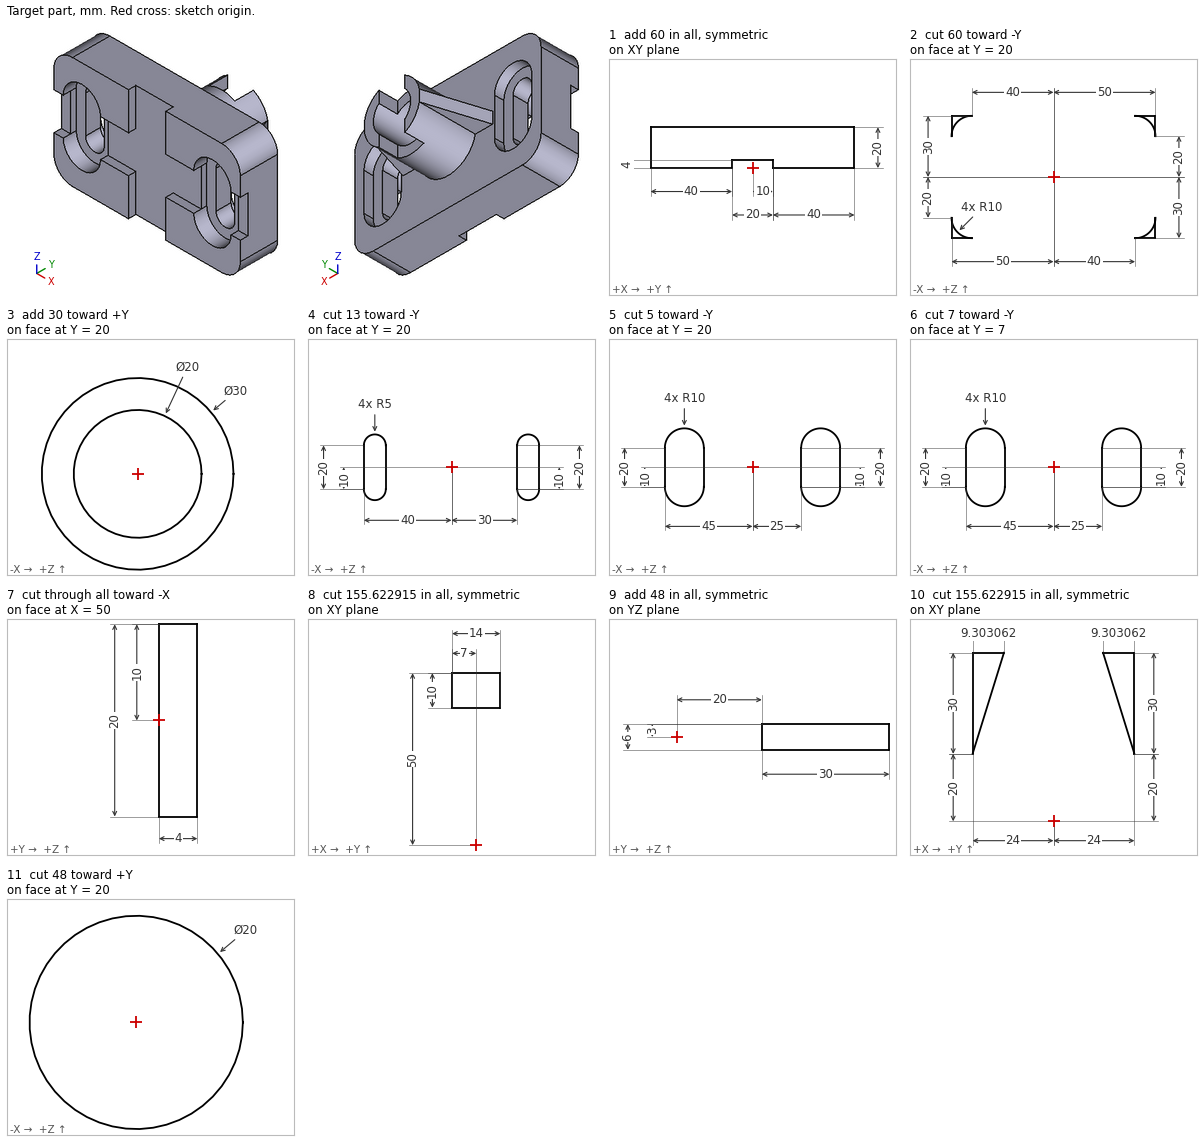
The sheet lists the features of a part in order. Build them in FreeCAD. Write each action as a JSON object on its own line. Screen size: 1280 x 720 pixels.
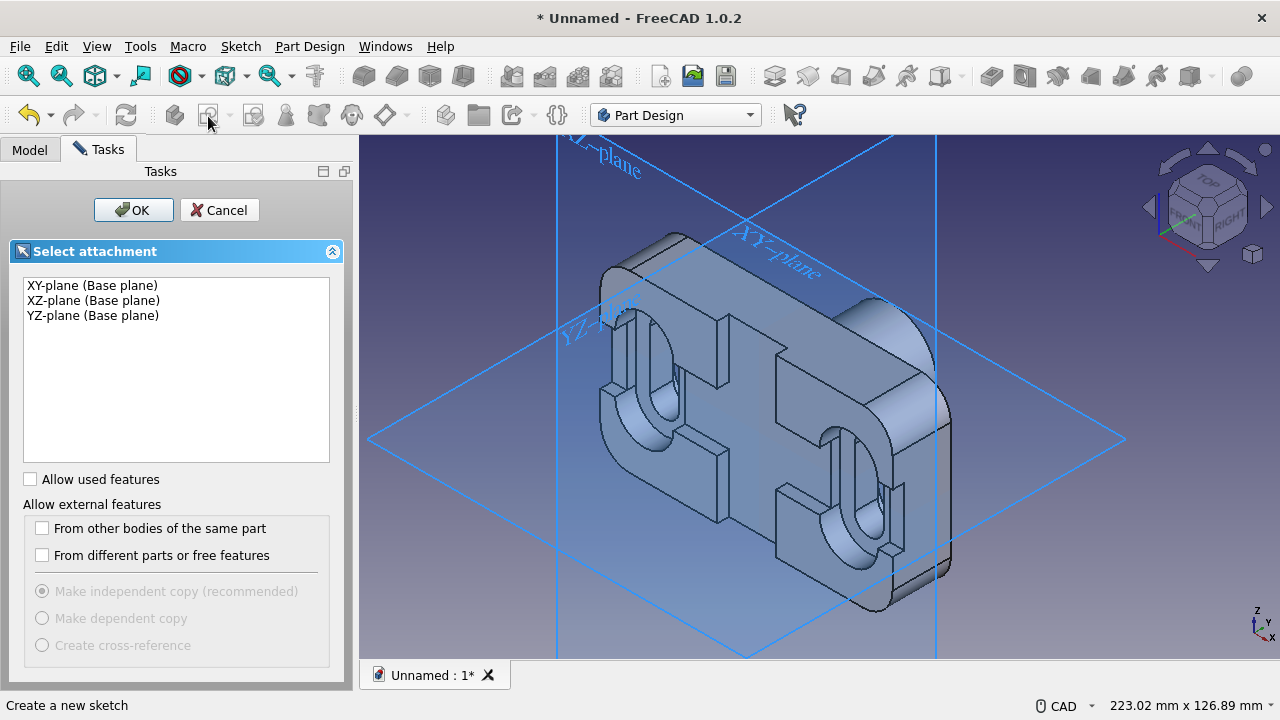
{"action": "left_click", "coordinate": [84, 286]}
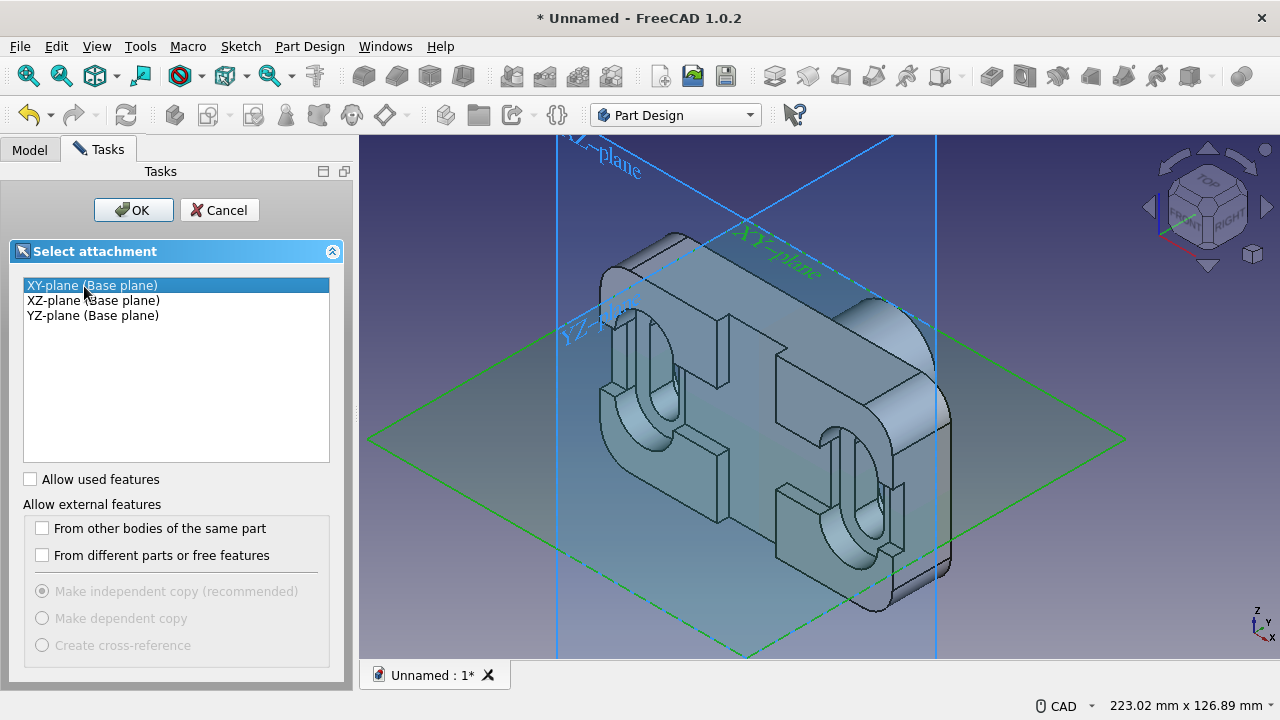
{"action": "left_click", "coordinate": [134, 210]}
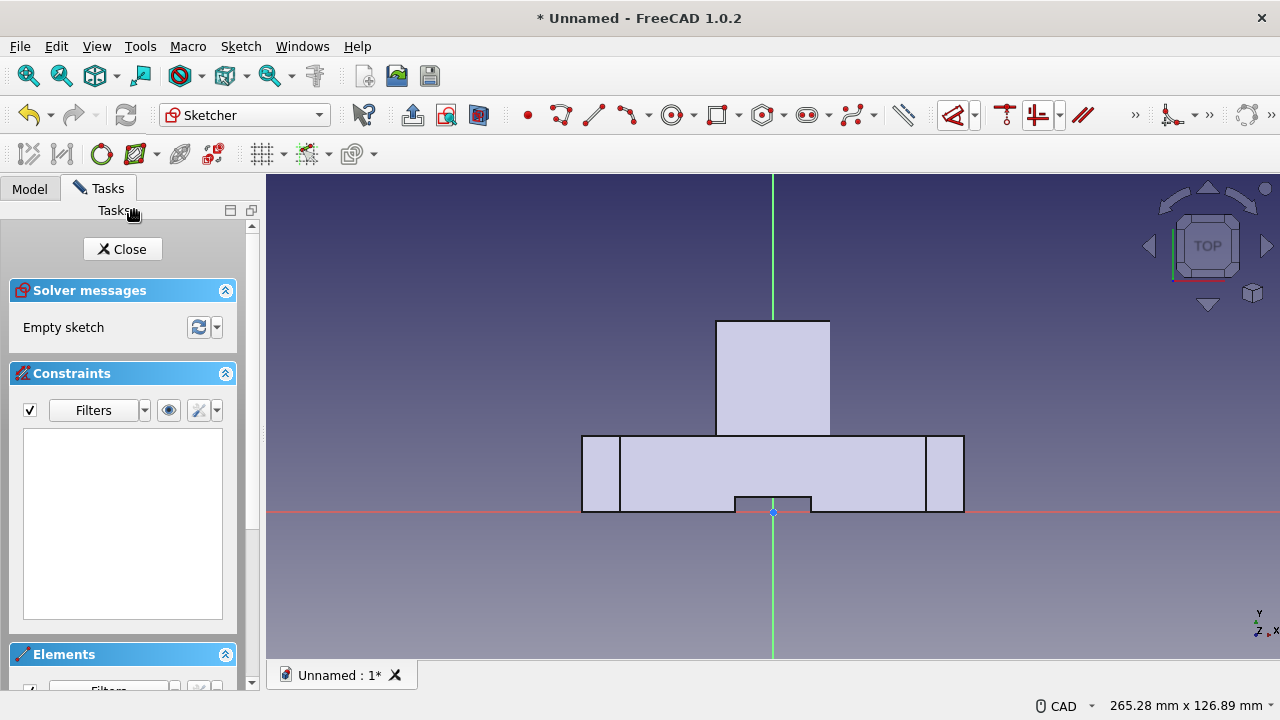
{"action": "left_click", "coordinate": [479, 116]}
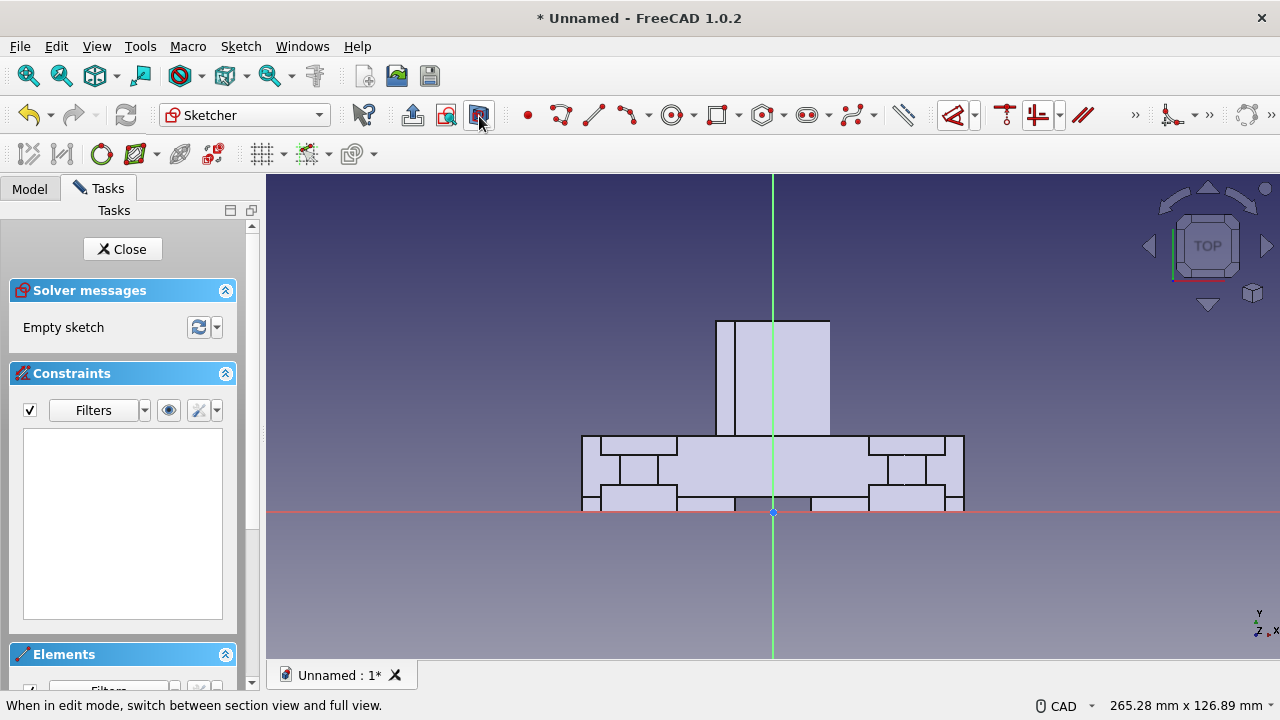
{"action": "scroll", "coordinate": [784, 328], "scroll_direction": "up", "scroll_amount": 10}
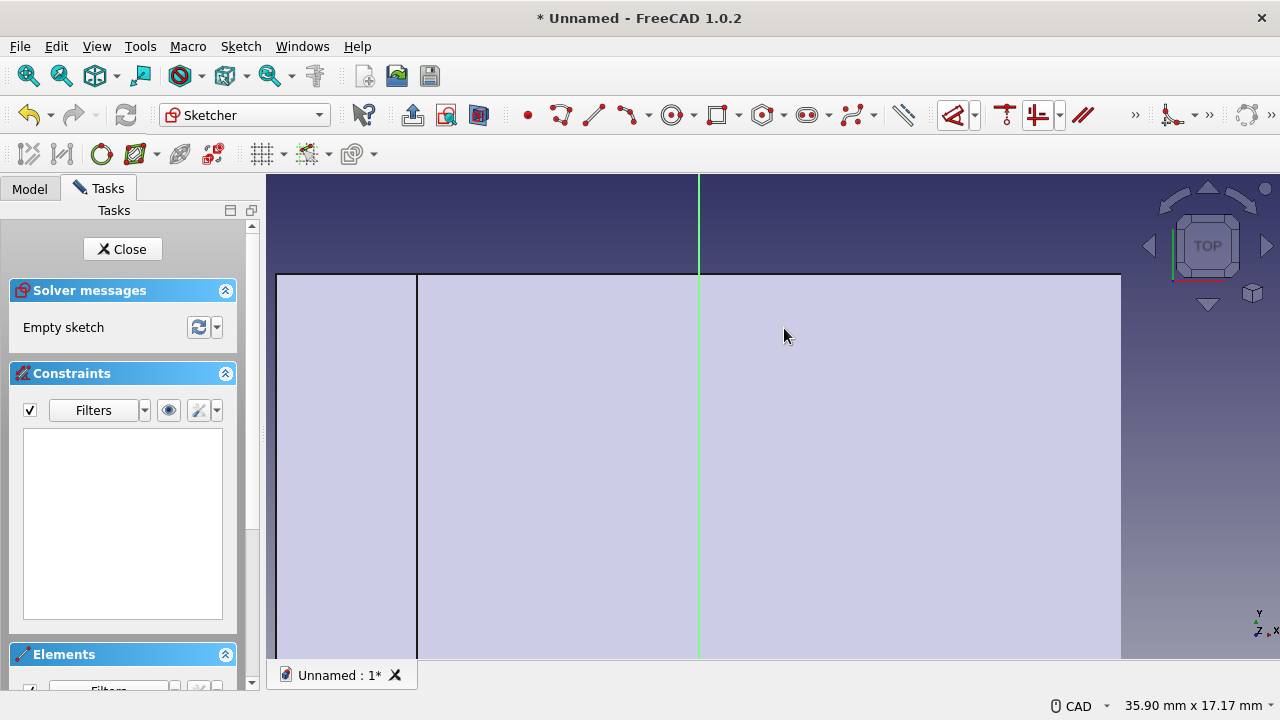
{"action": "key", "text": "g r"}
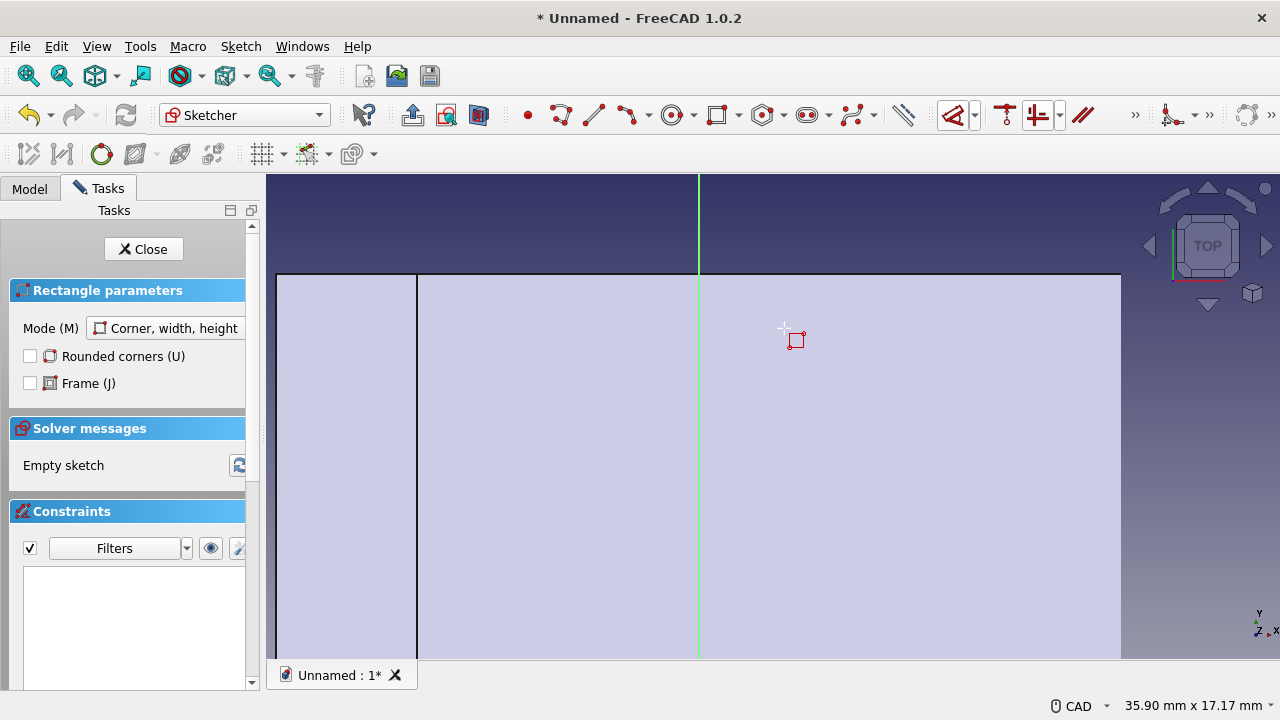
{"action": "left_click", "coordinate": [502, 274]}
{"action": "left_click", "coordinate": [897, 556]}
{"action": "key", "text": "Escape"}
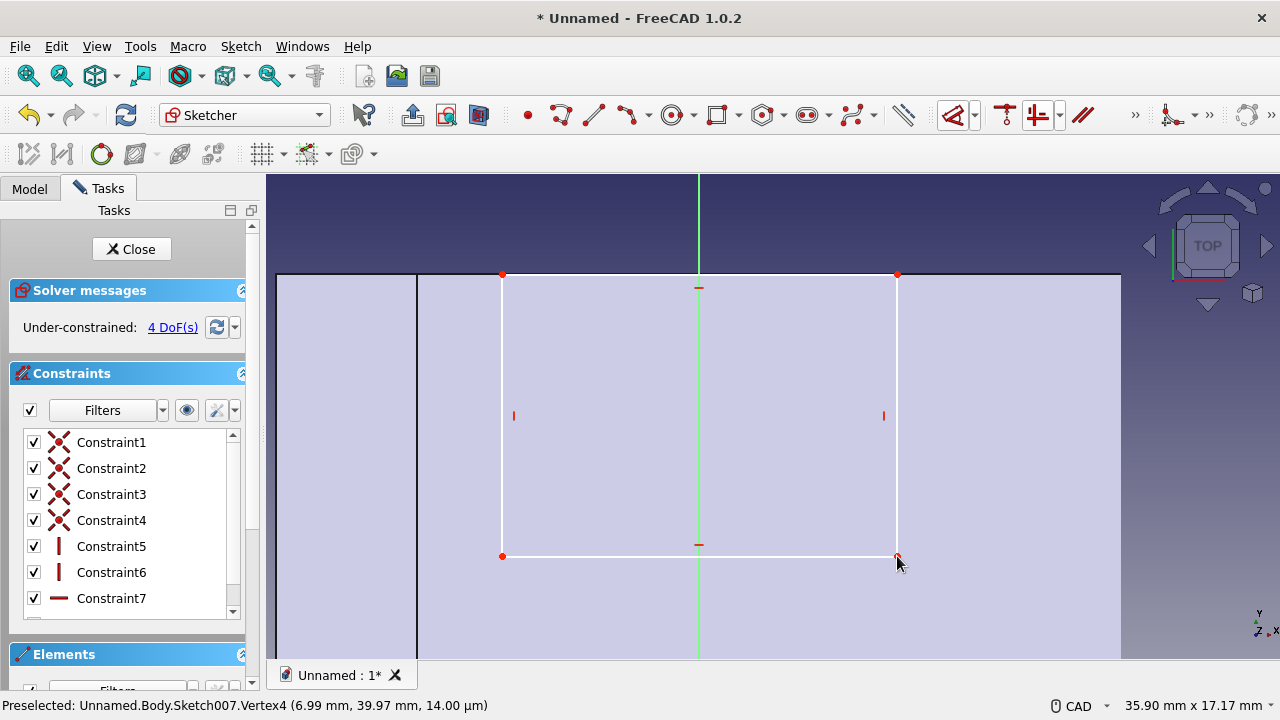
{"action": "left_click", "coordinate": [502, 360]}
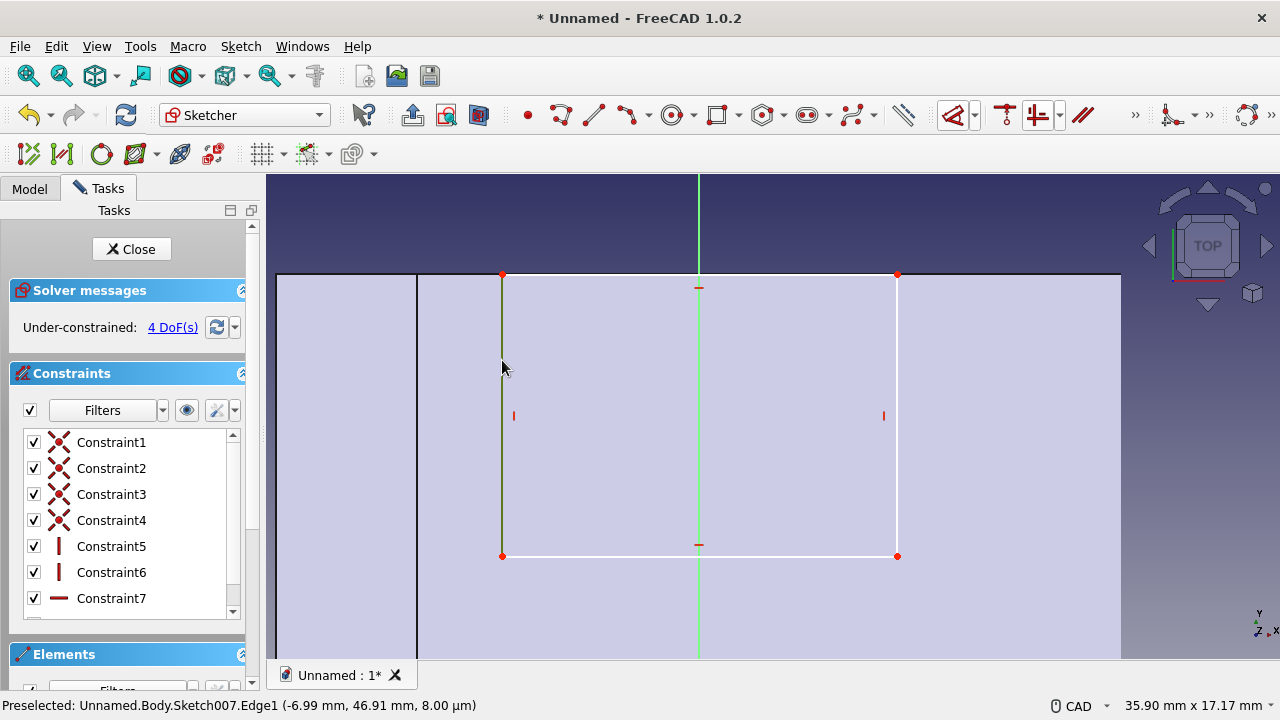
{"action": "left_click", "coordinate": [974, 116]}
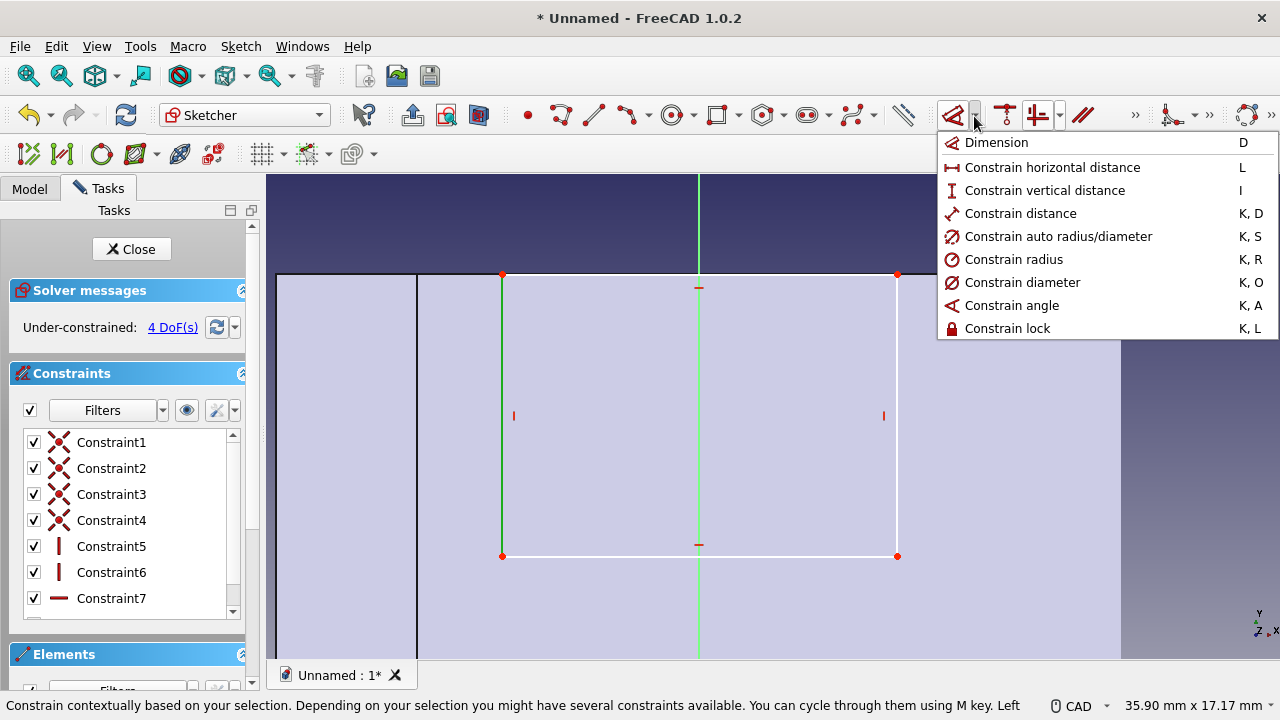
{"action": "left_click", "coordinate": [1108, 190]}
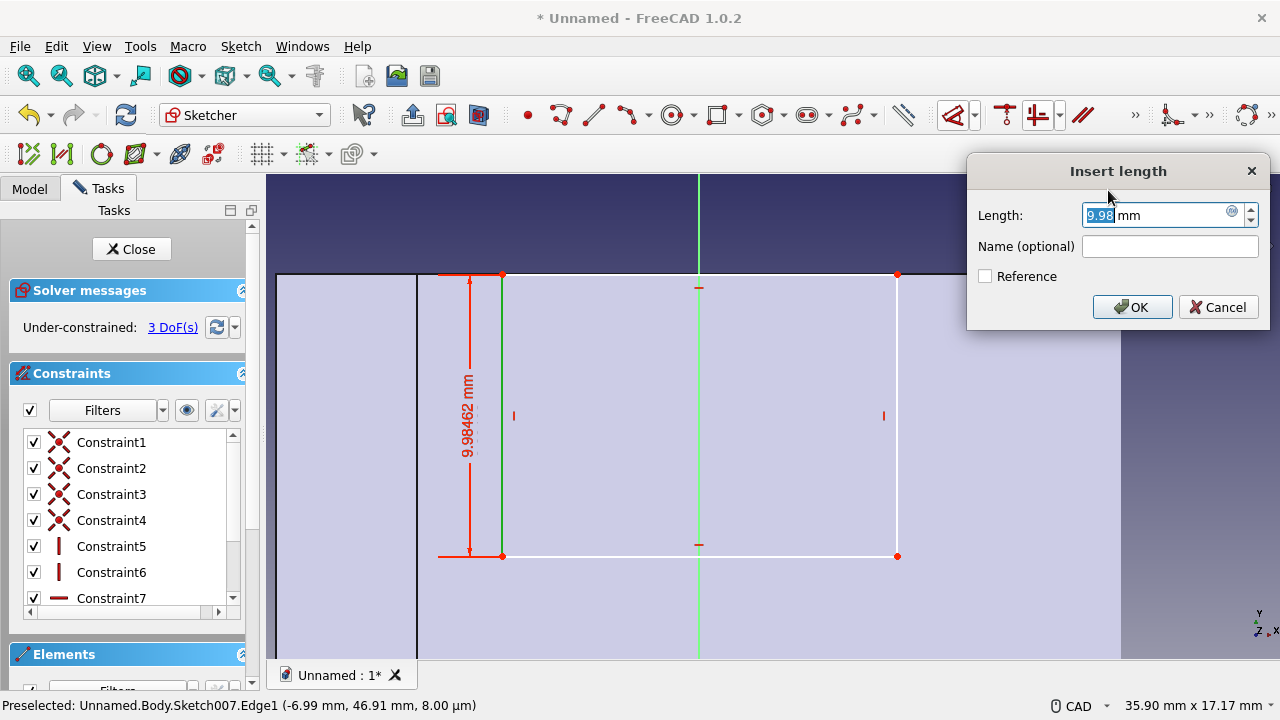
{"action": "type", "text": "10"}
{"action": "key", "text": "Return"}